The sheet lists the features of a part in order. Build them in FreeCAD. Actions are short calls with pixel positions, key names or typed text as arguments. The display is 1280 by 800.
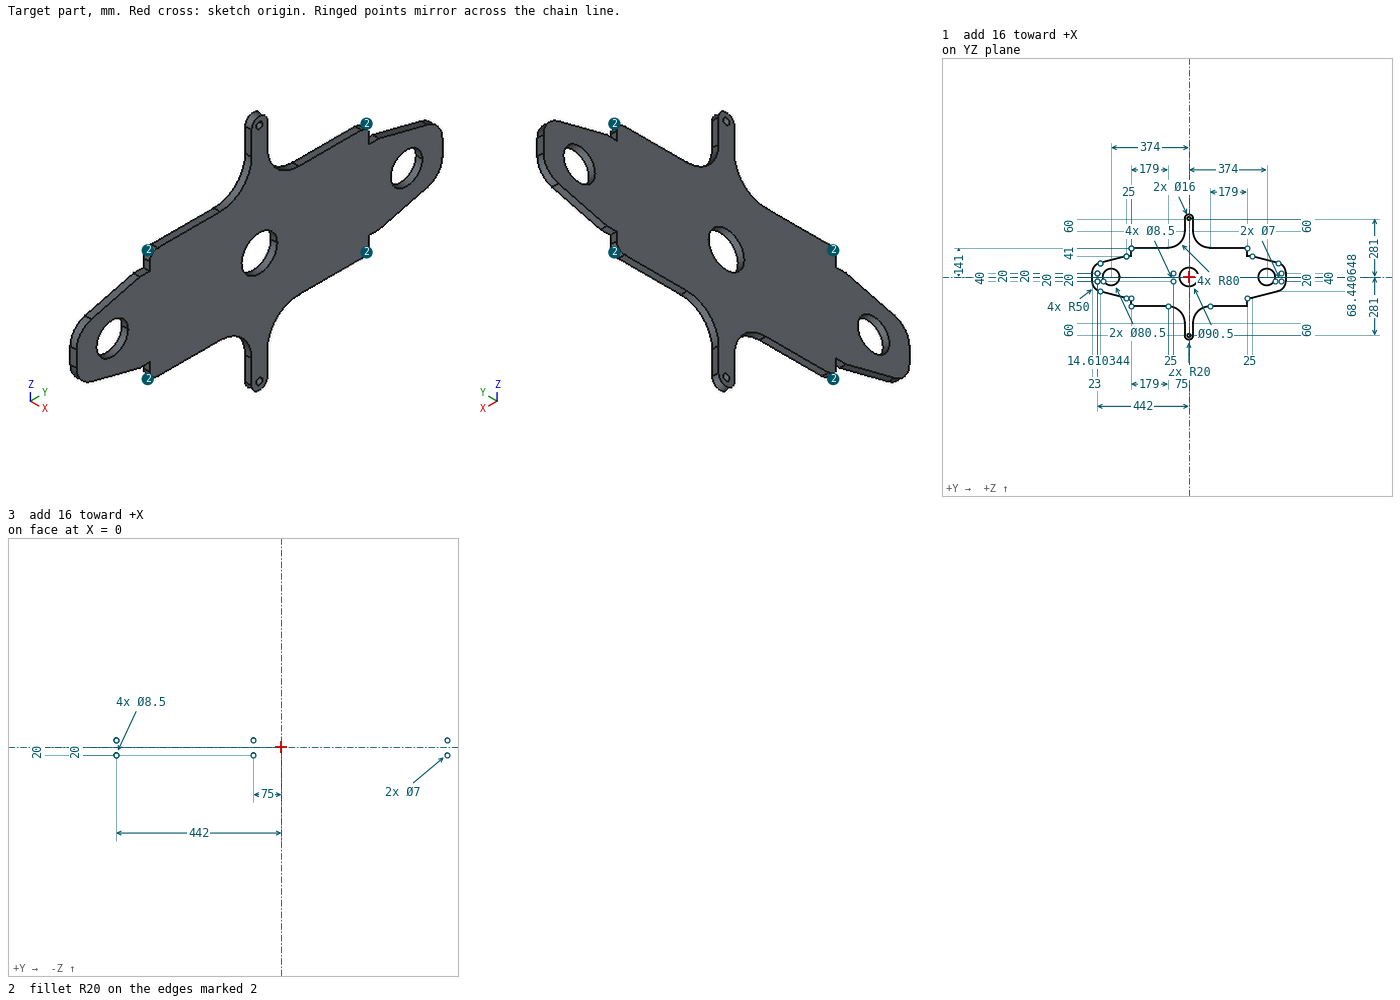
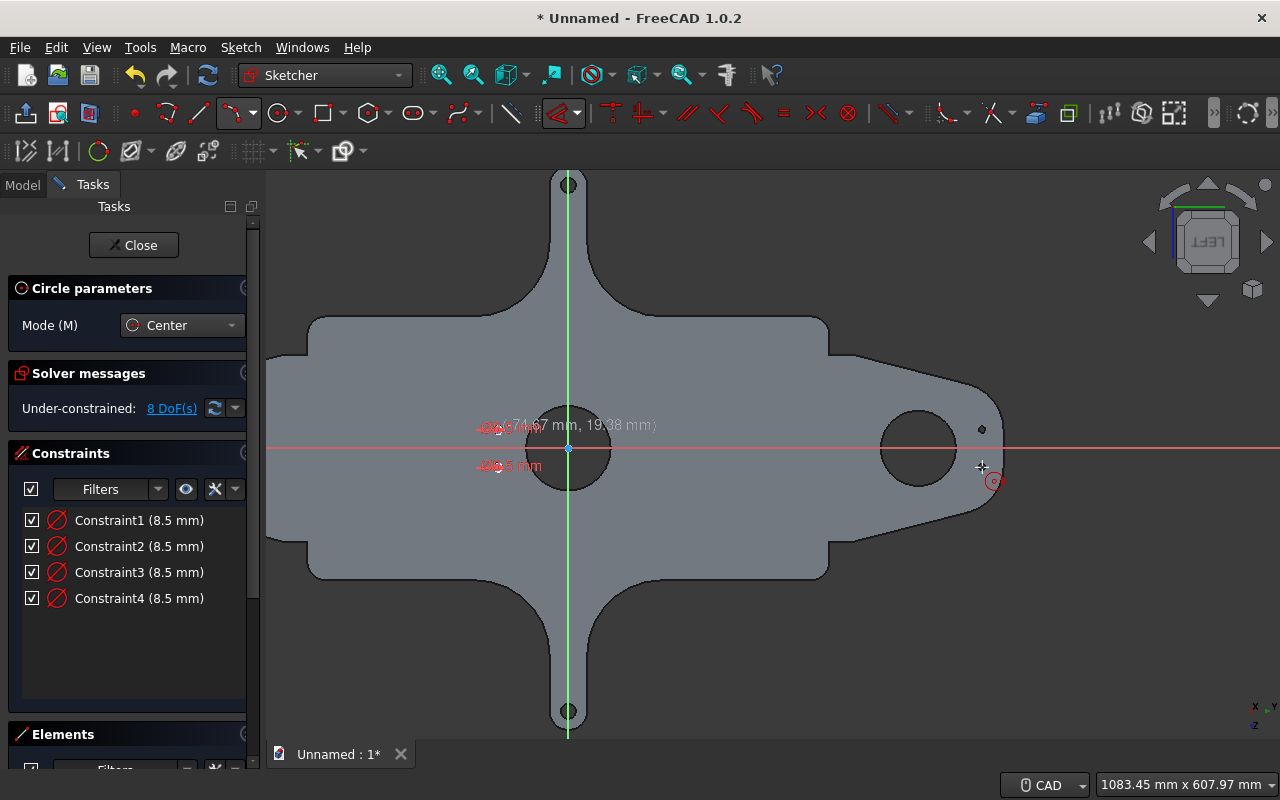
click(982, 467)
move(984, 465)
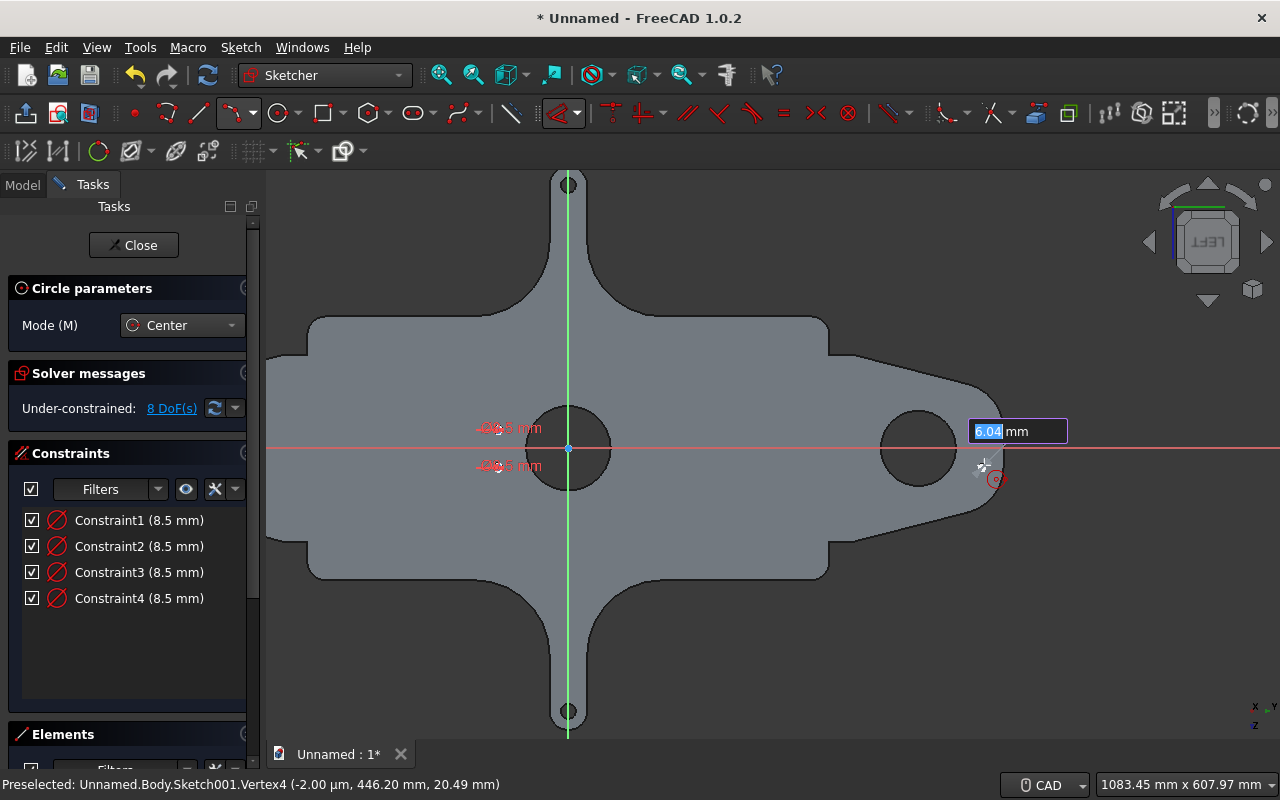
text(7)
key(Return)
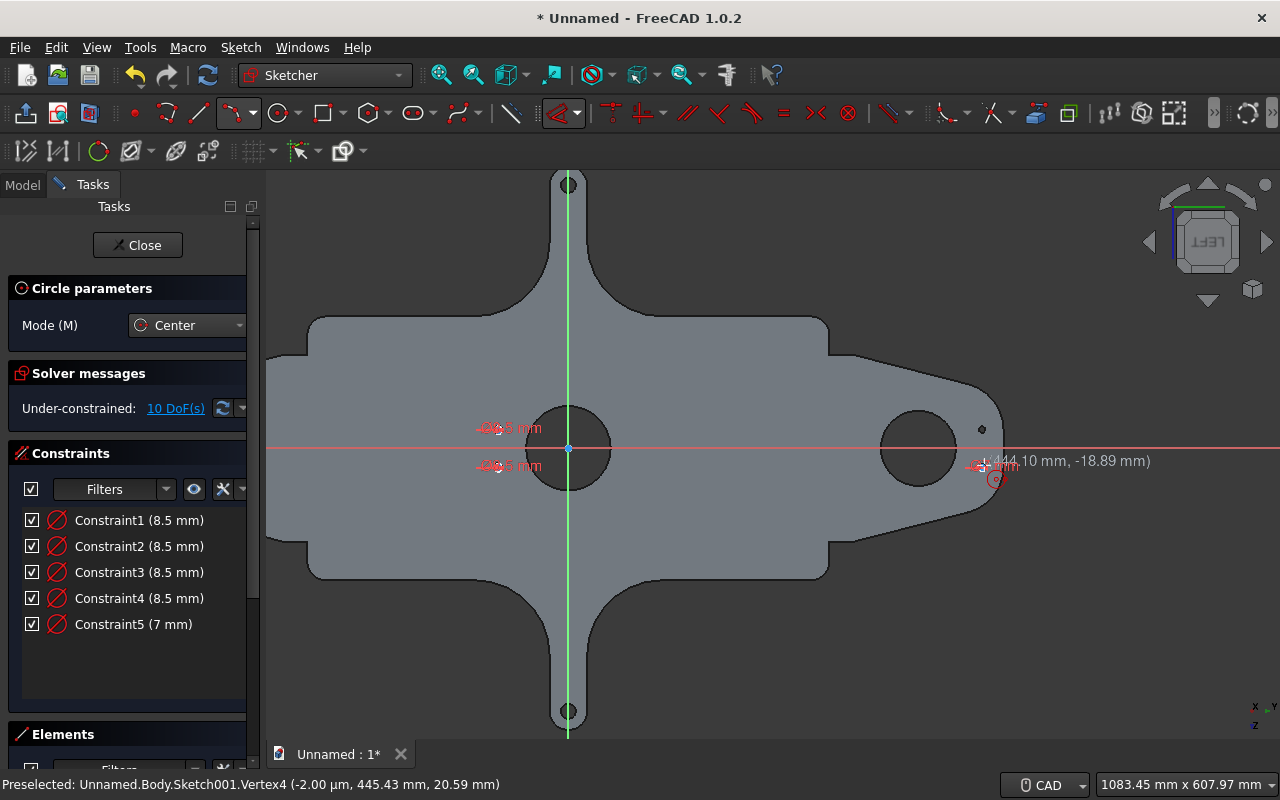
scroll(982, 430, up, 10)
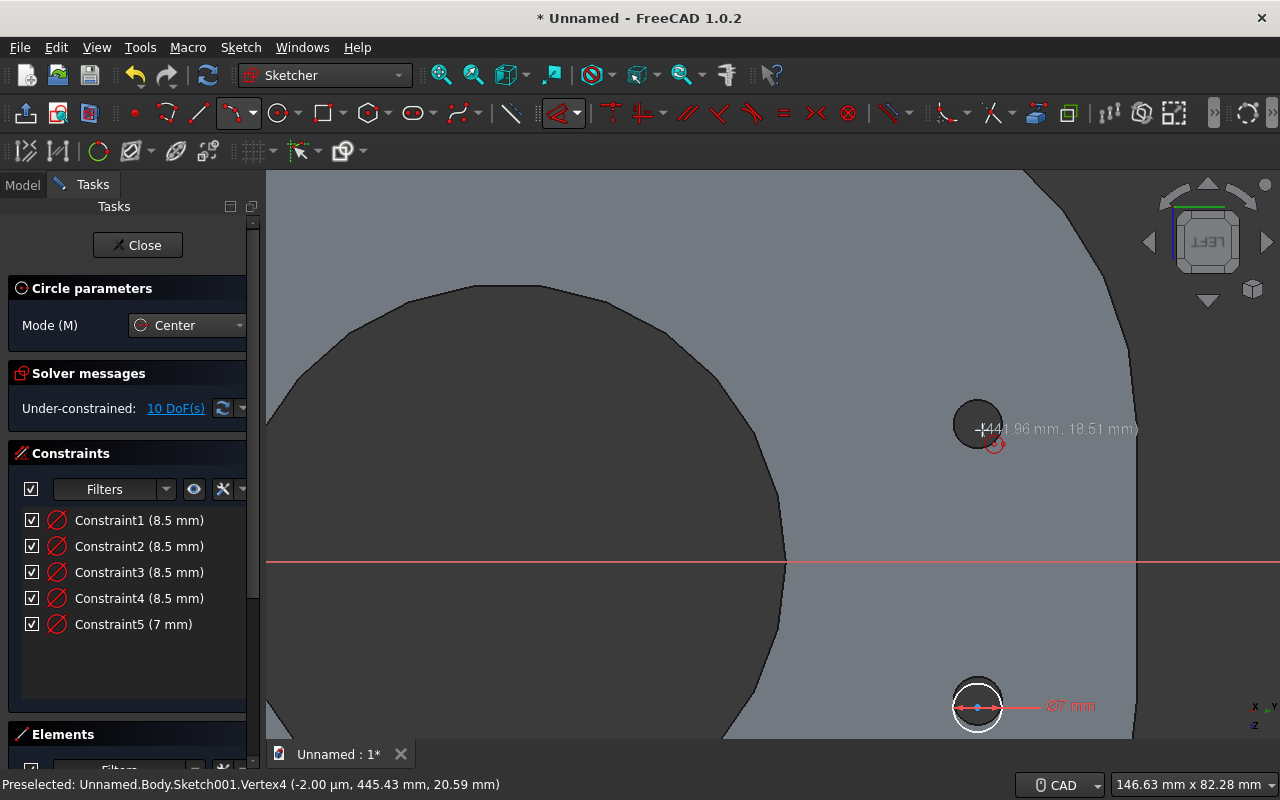
scroll(982, 444, down, 12)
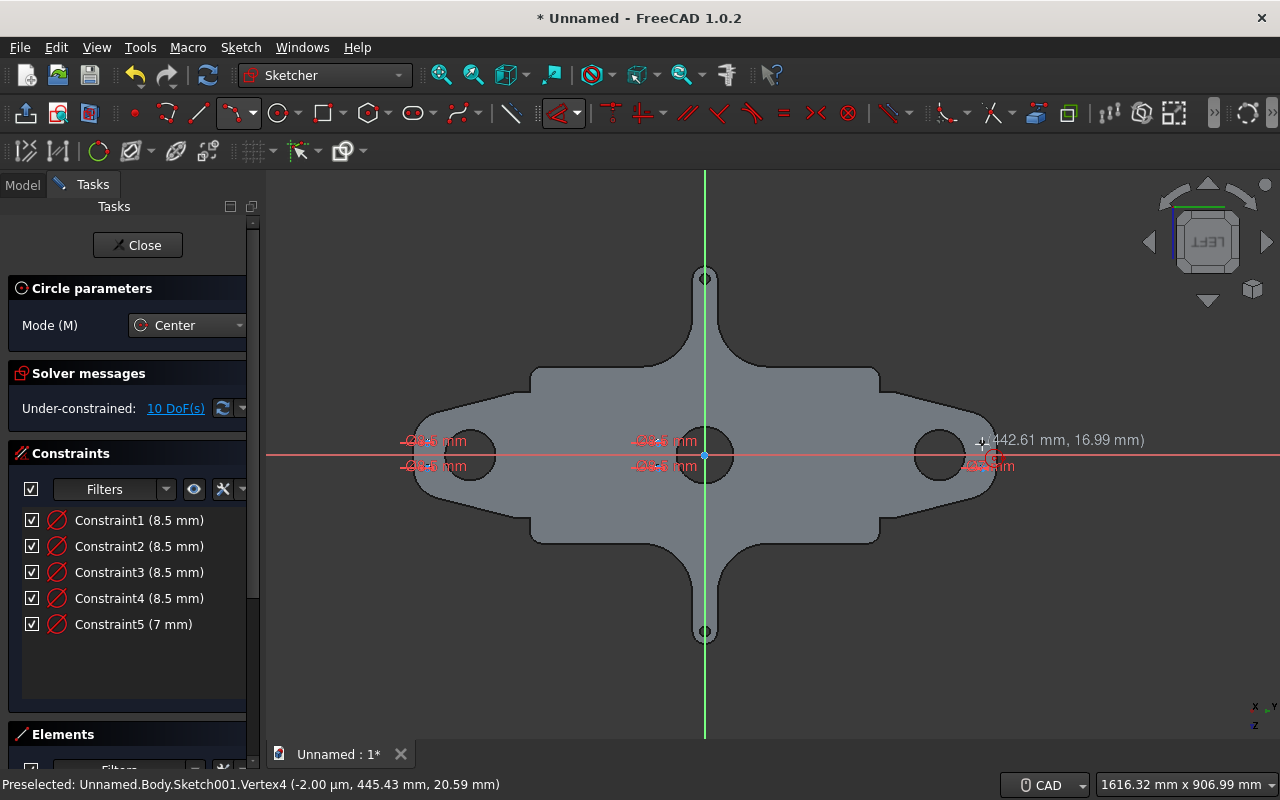
scroll(982, 443, up, 2)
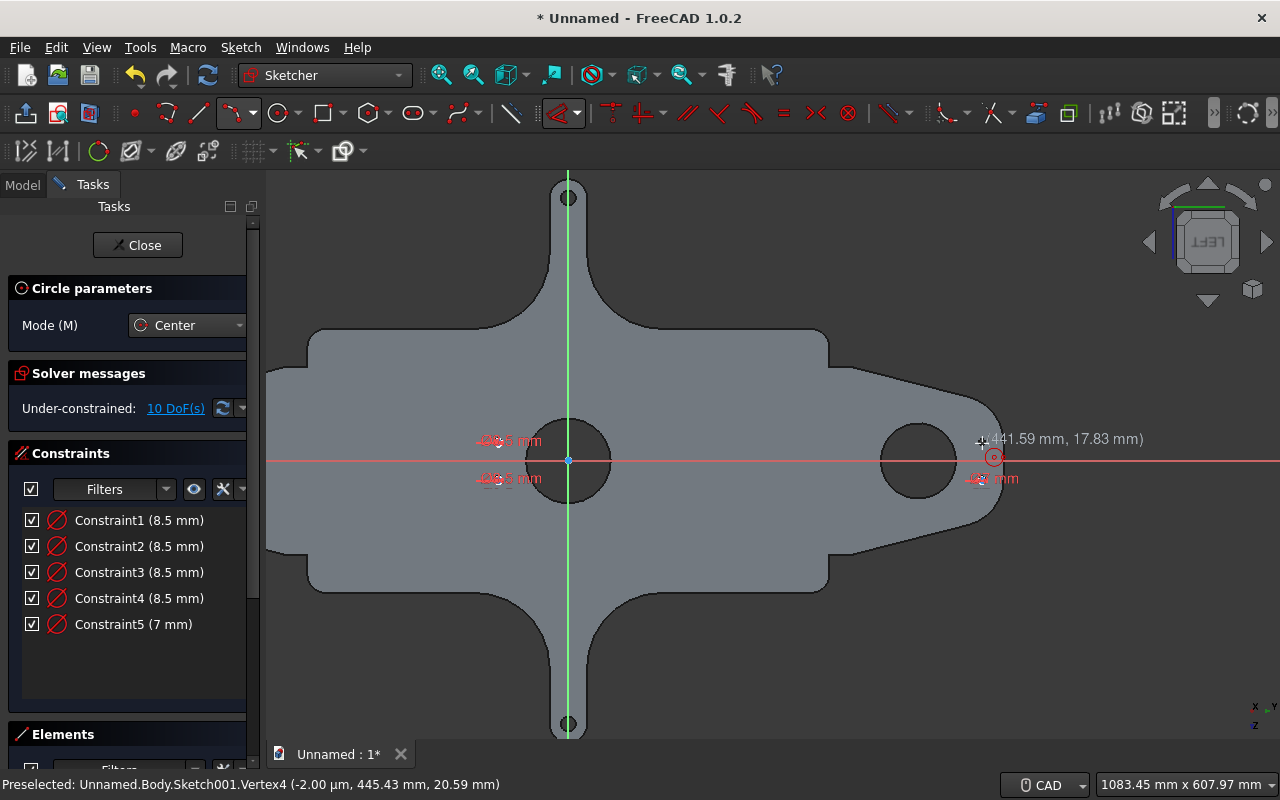
click(982, 442)
move(984, 440)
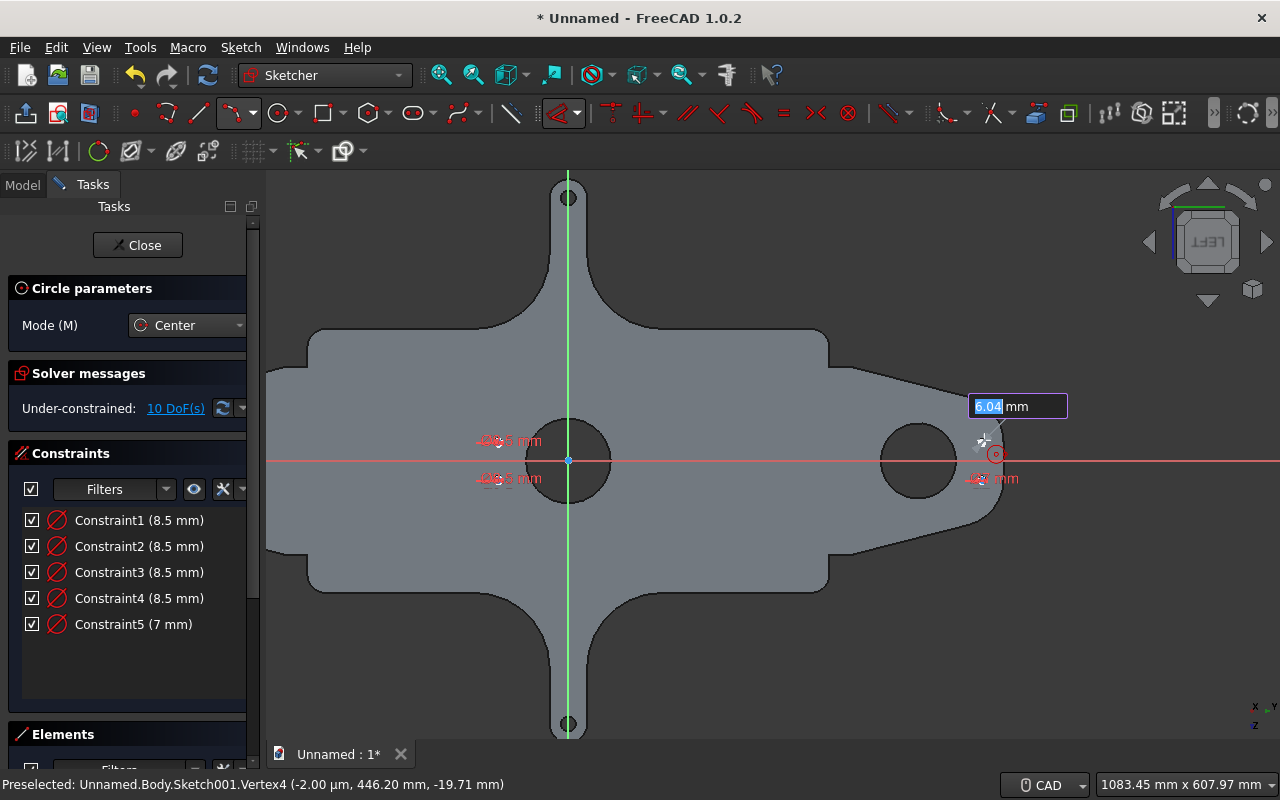
text(7)
key(Return)
key(Escape)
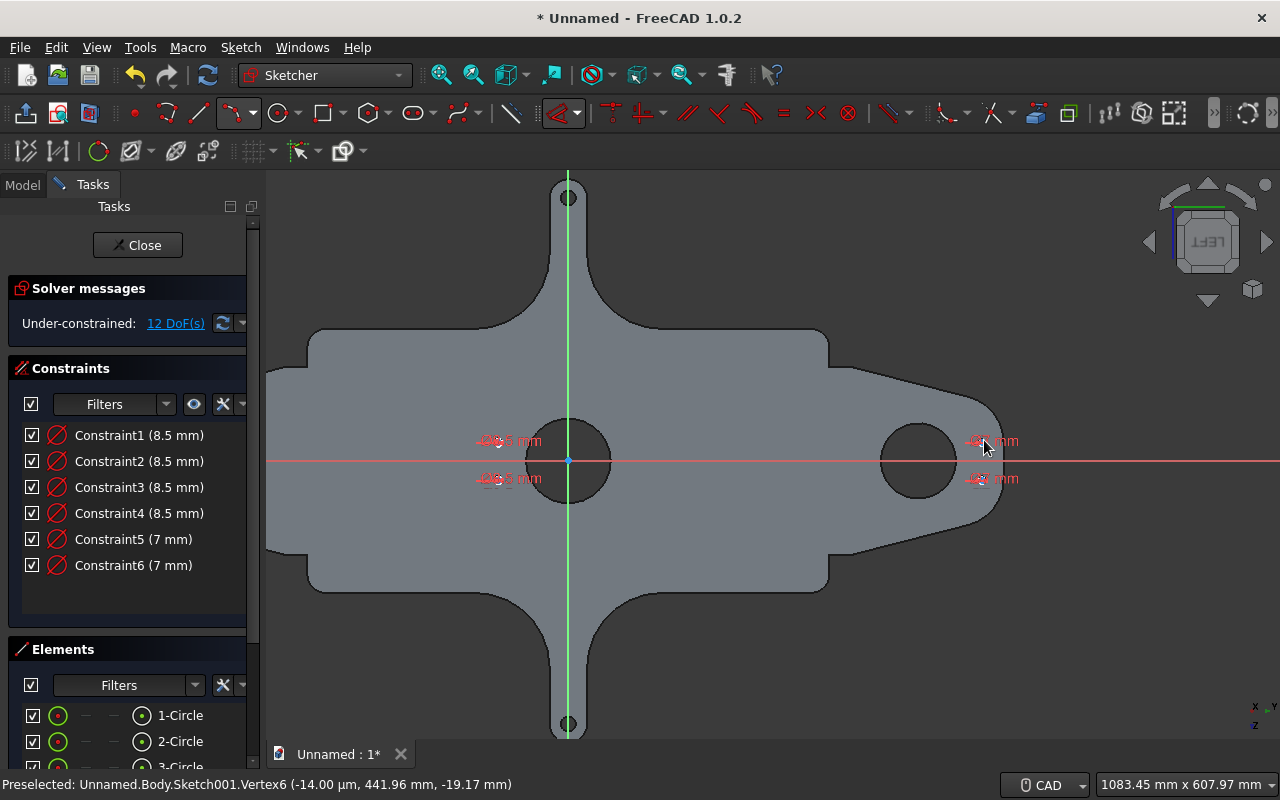
scroll(982, 441, down, 2)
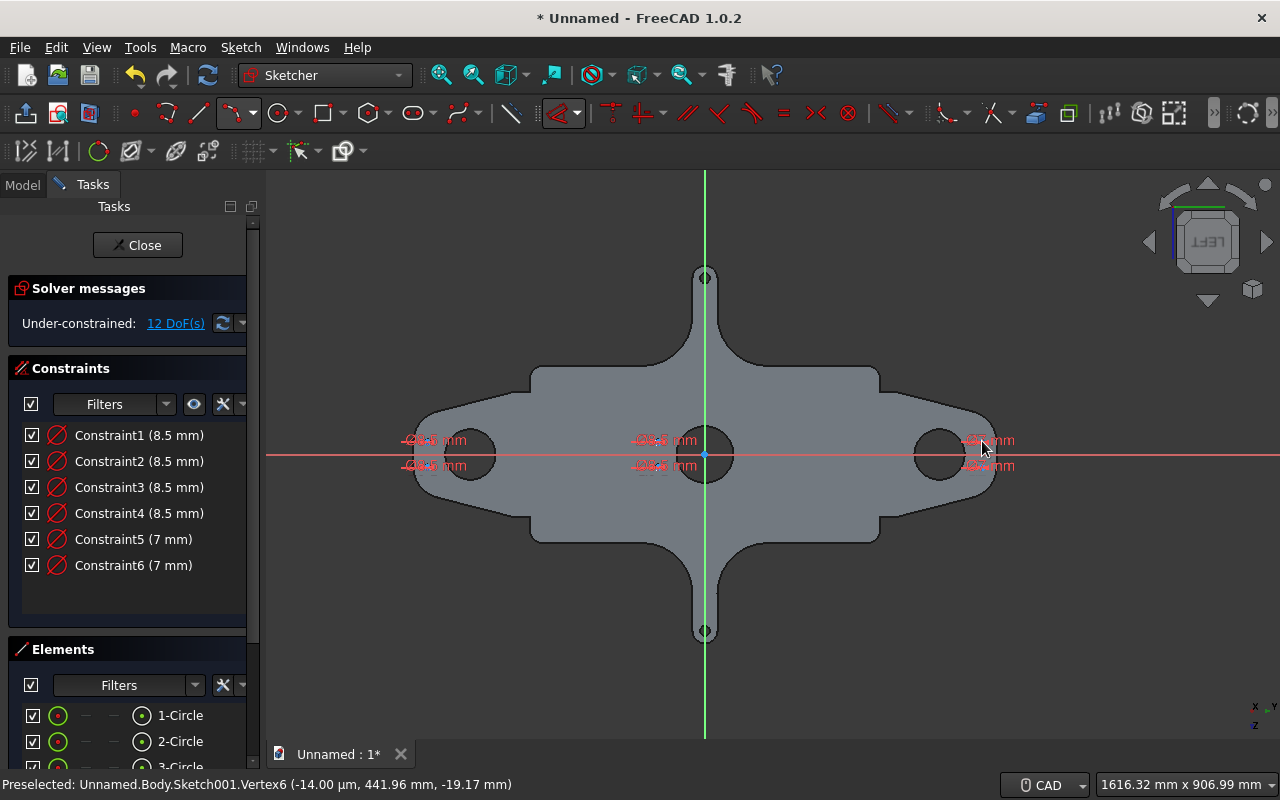
click(428, 468)